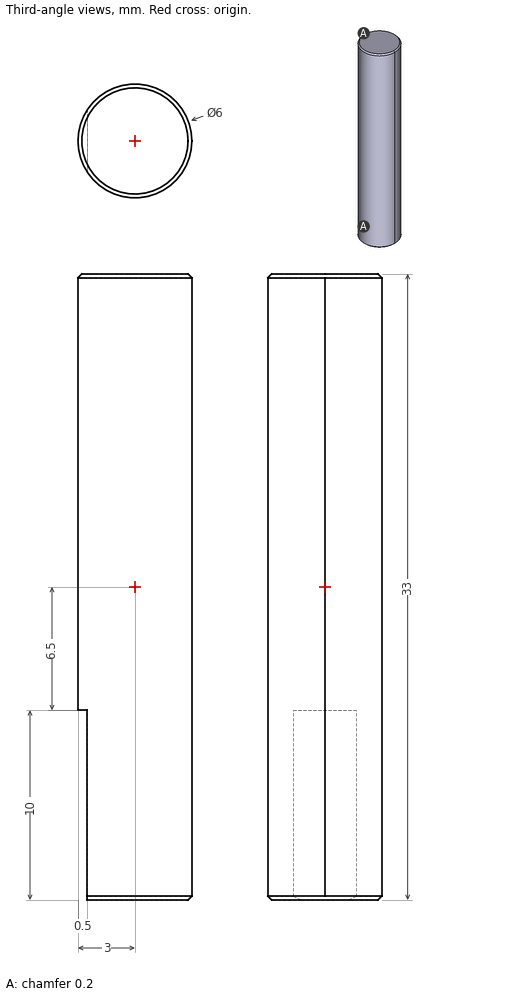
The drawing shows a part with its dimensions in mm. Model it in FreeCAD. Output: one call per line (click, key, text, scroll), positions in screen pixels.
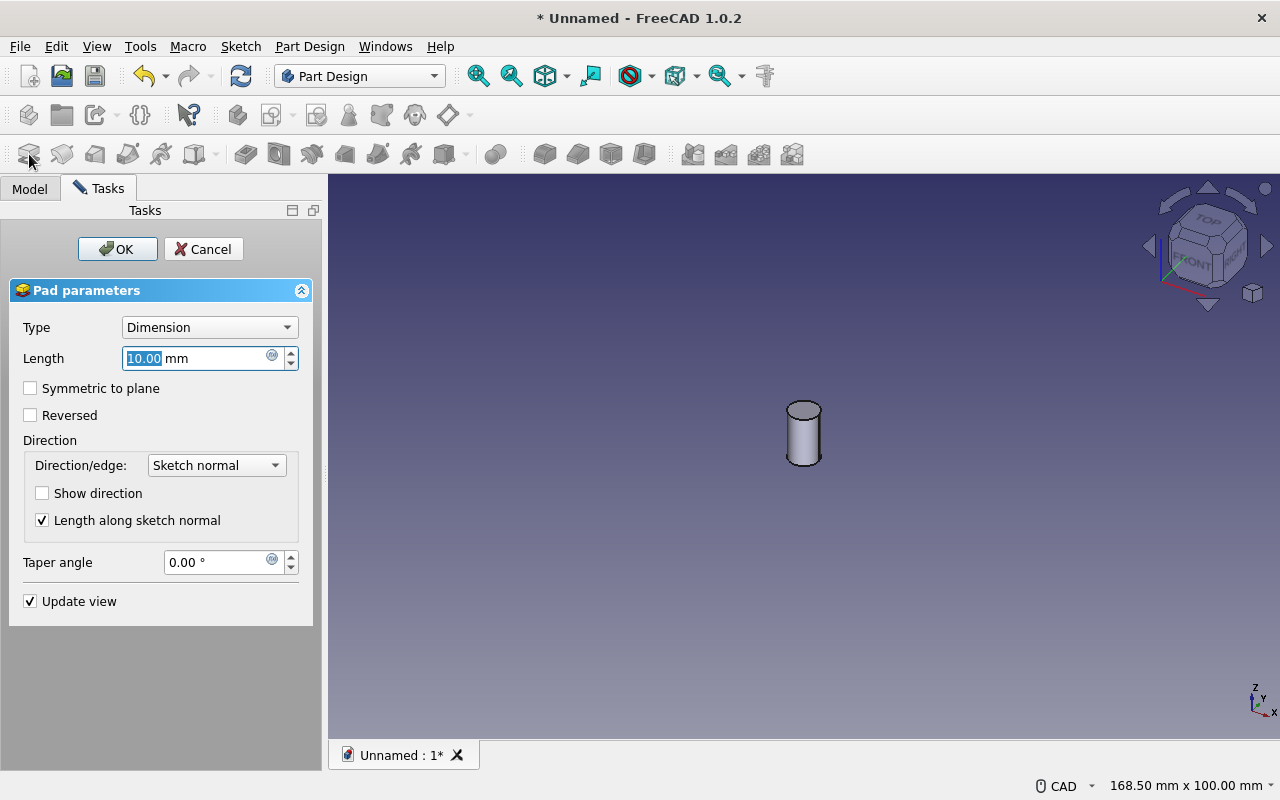
text(33)
key(Tab)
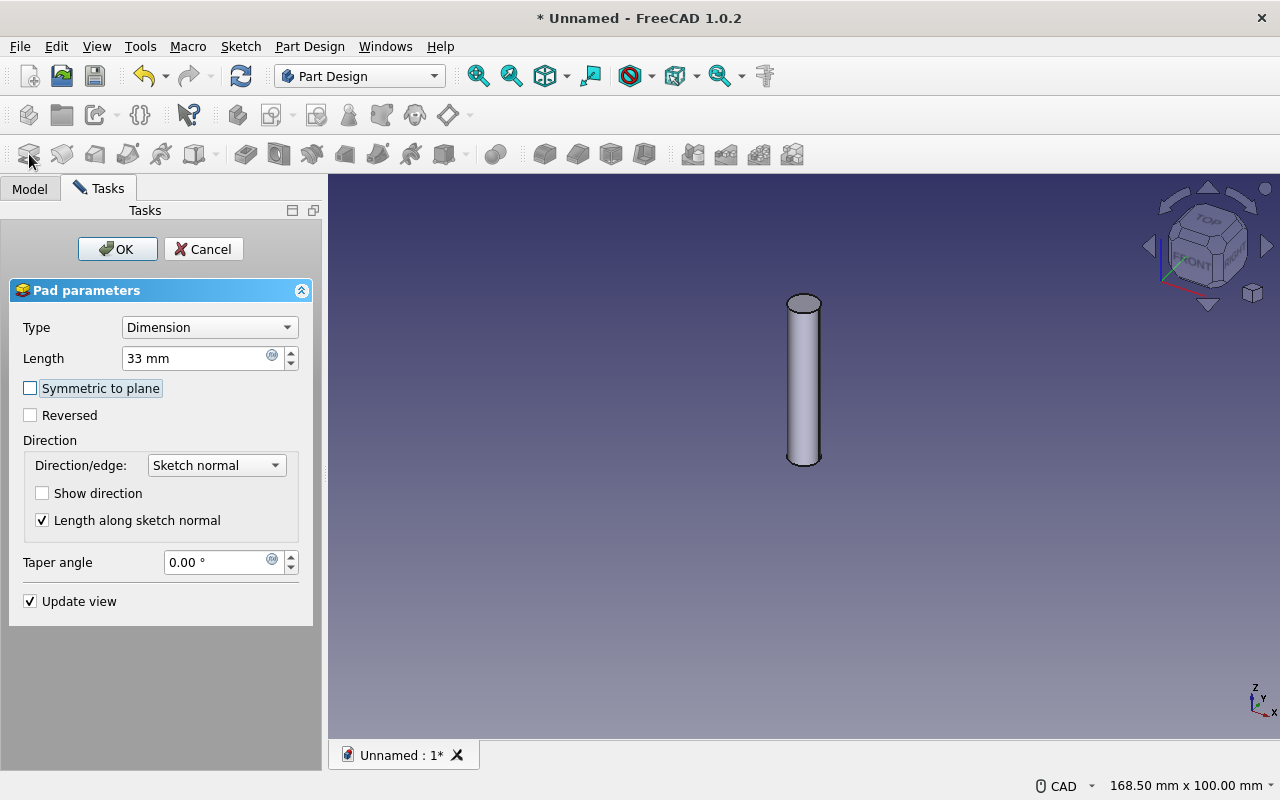
click(31, 388)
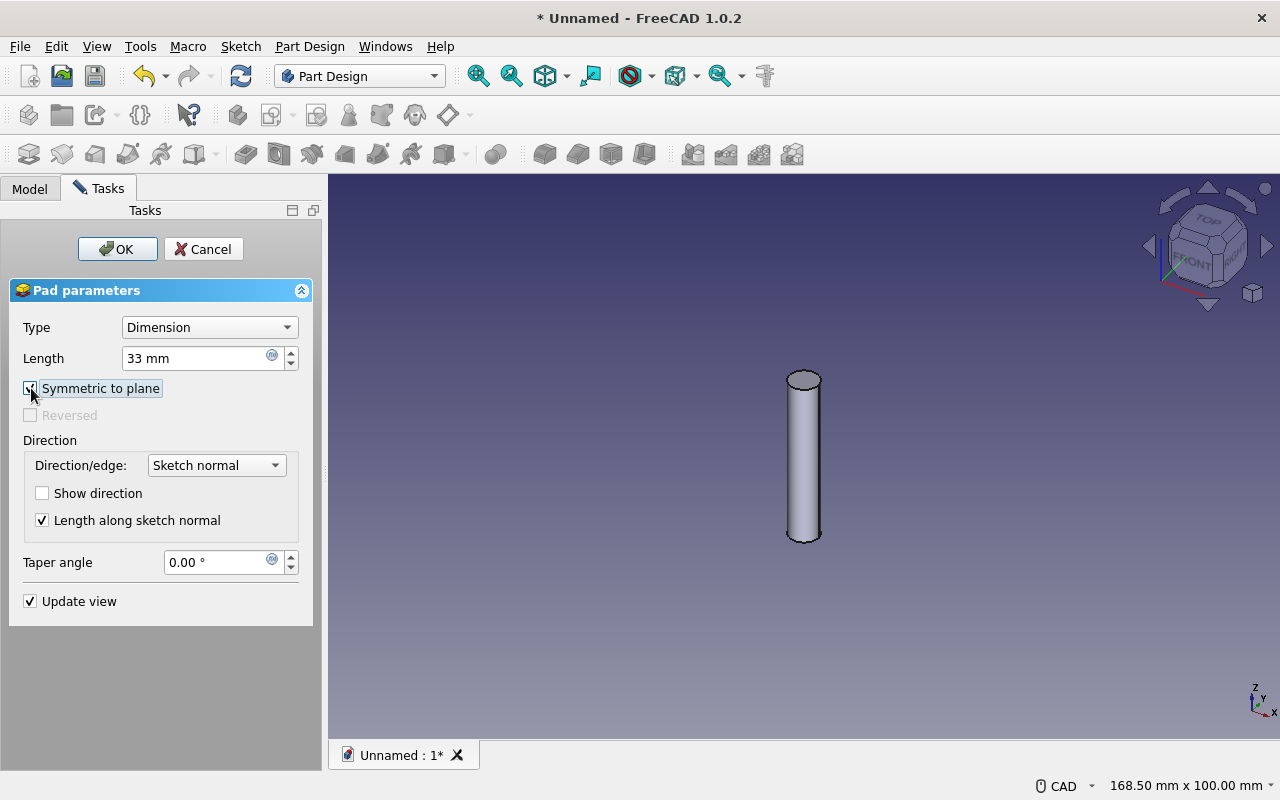
click(118, 249)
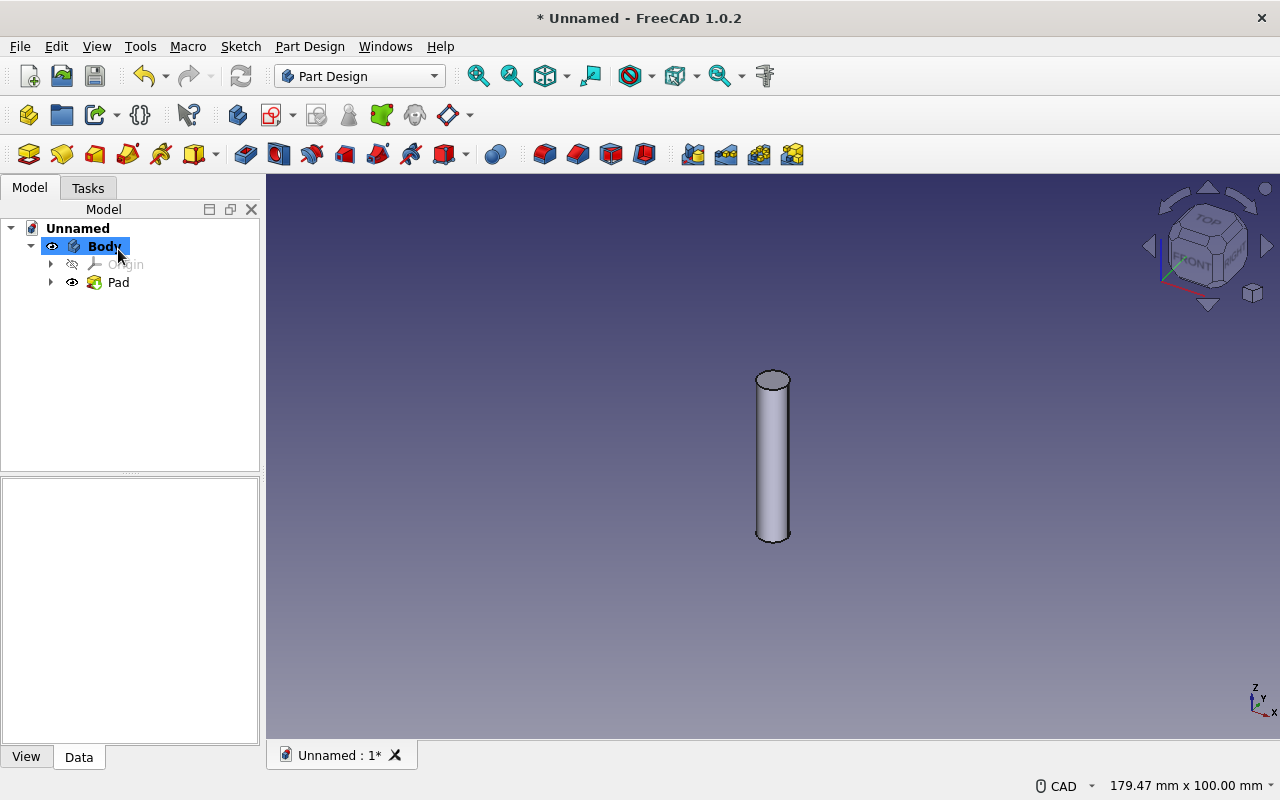
click(479, 76)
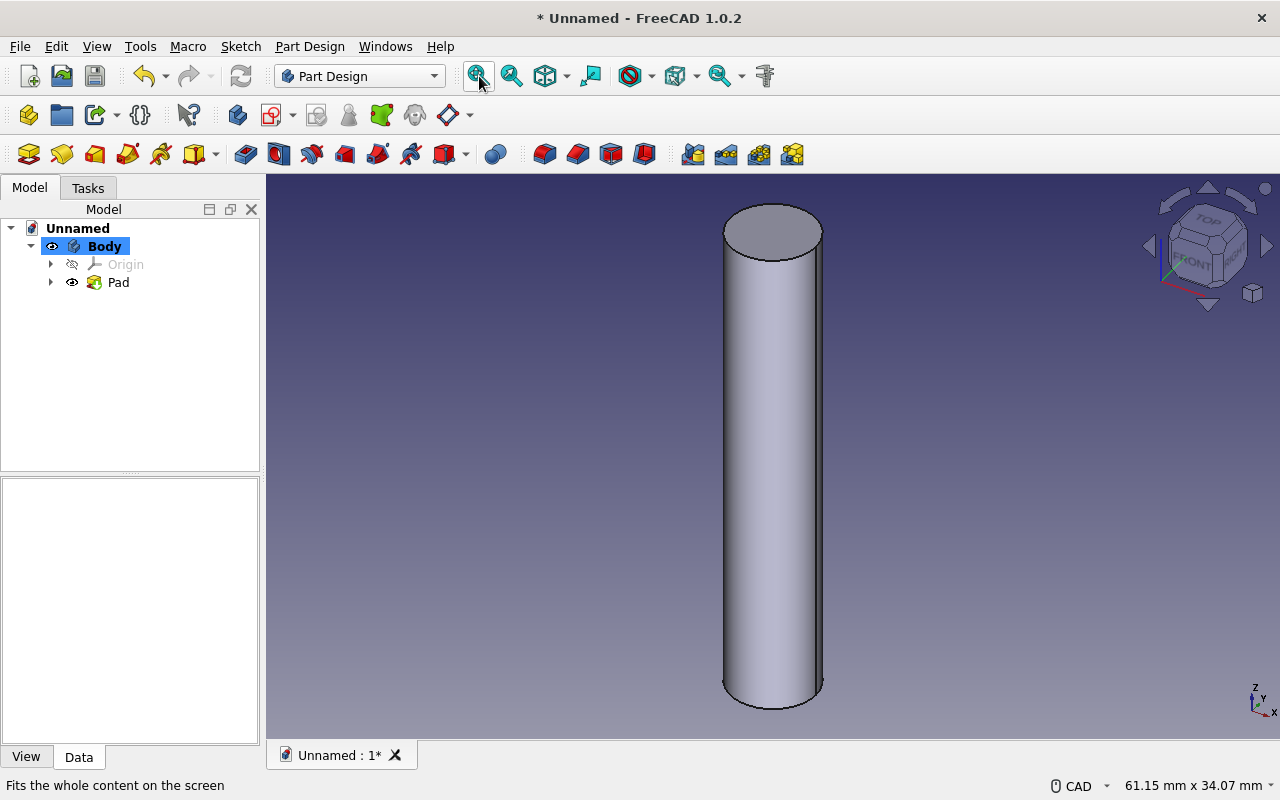
click(736, 699)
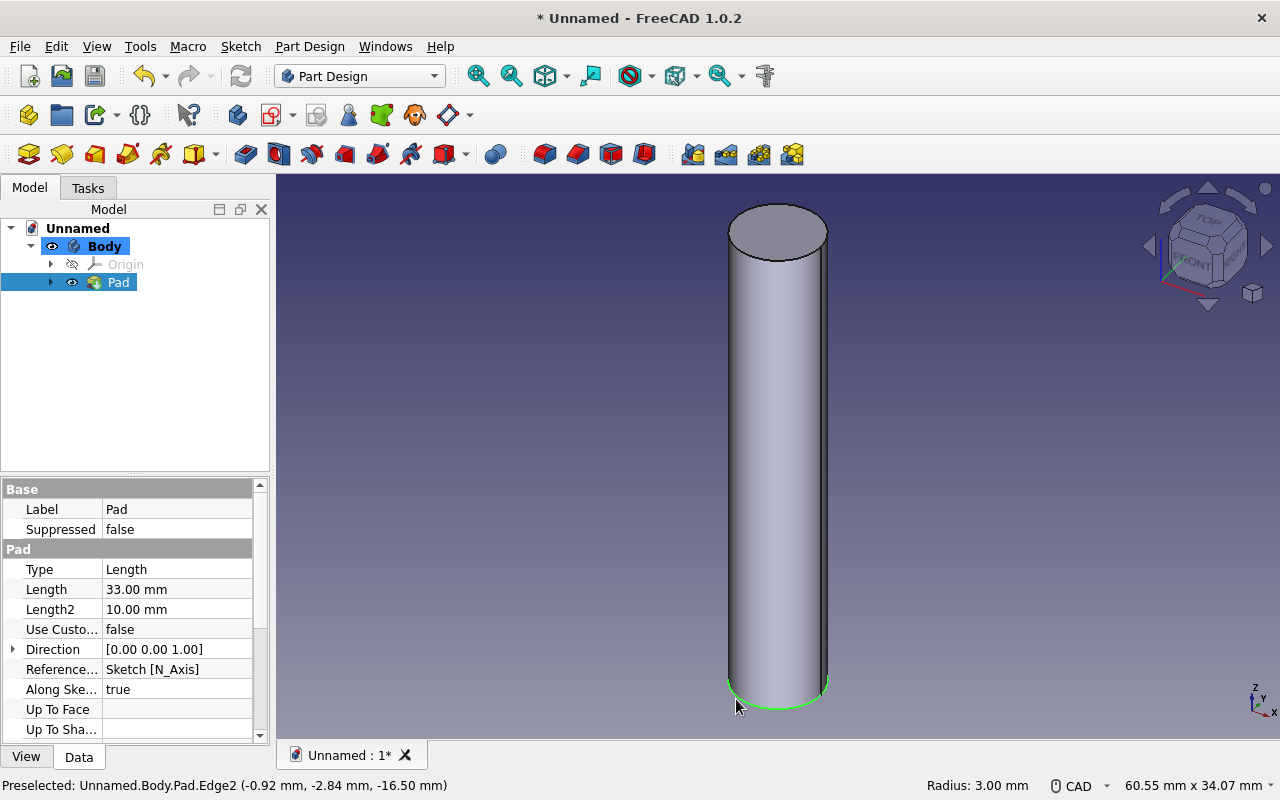
click(729, 234, ctrl)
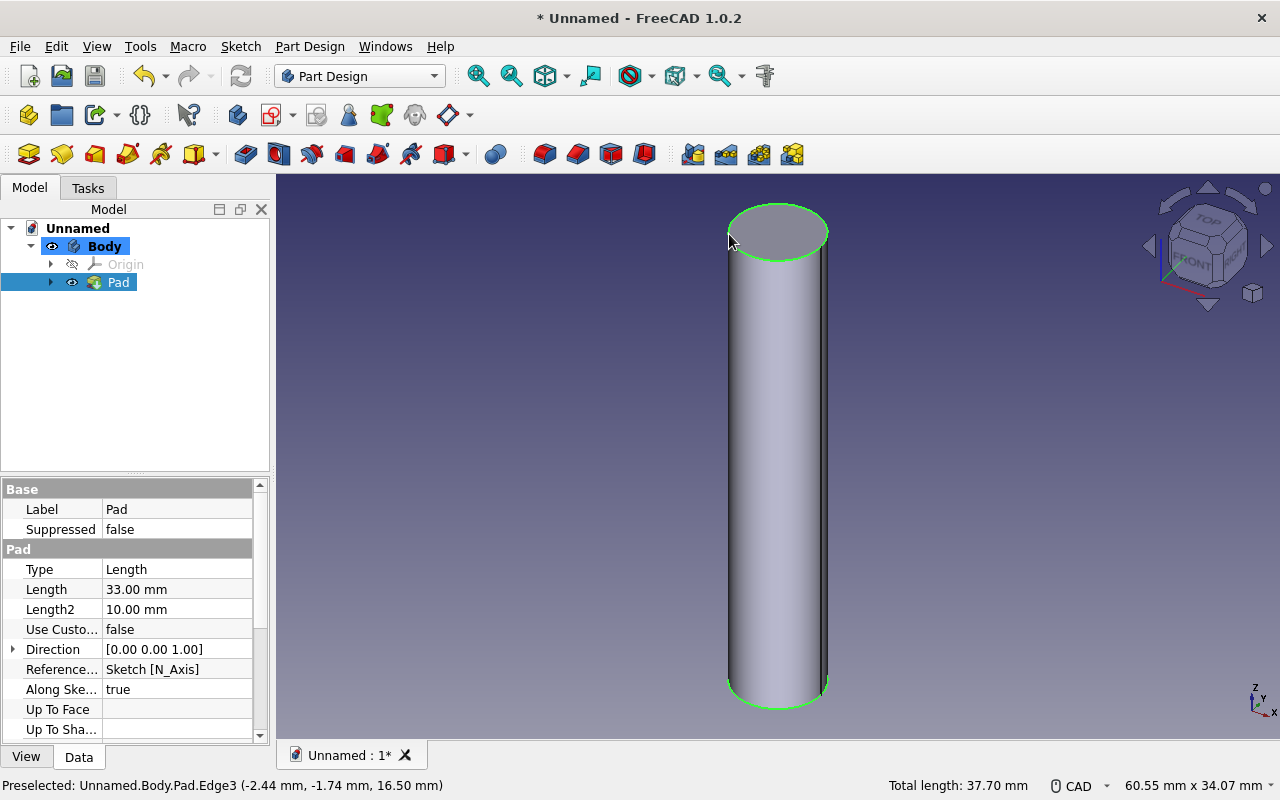
click(578, 154)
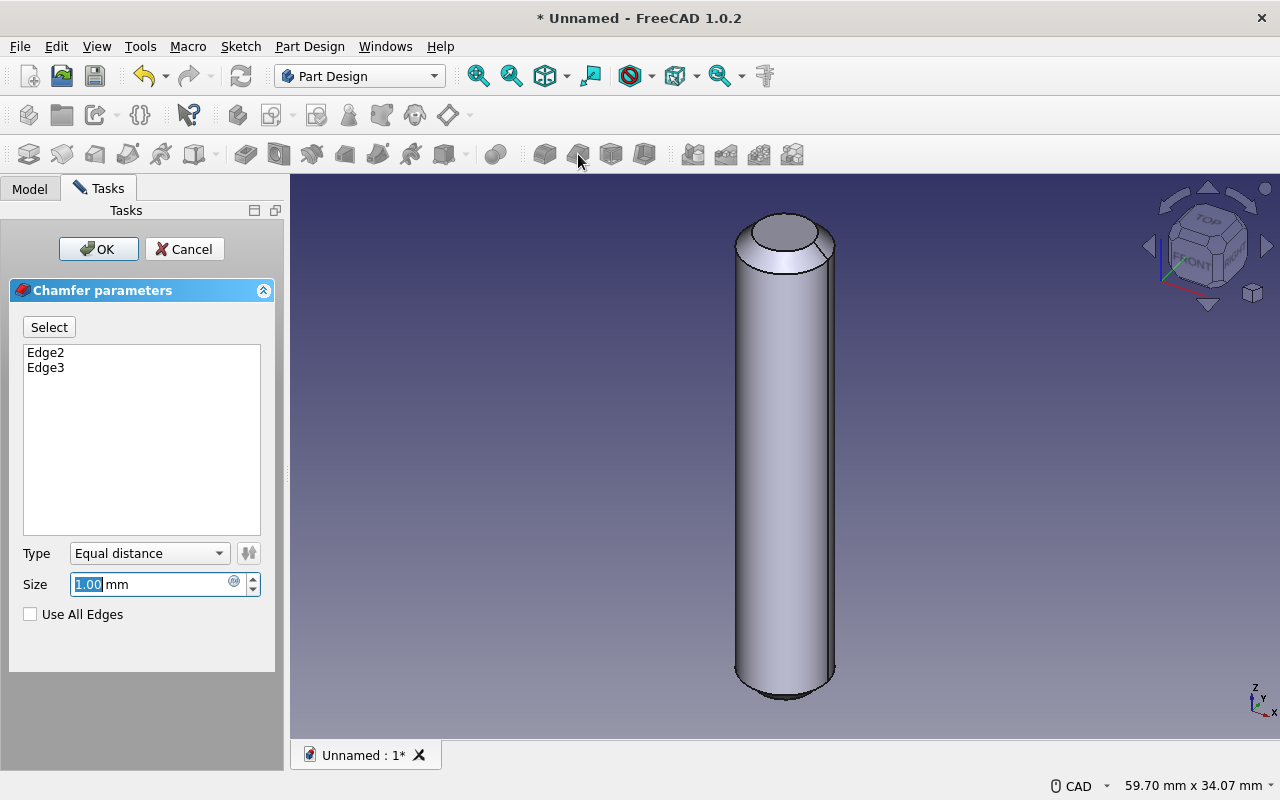
text(0.2)
key(Tab)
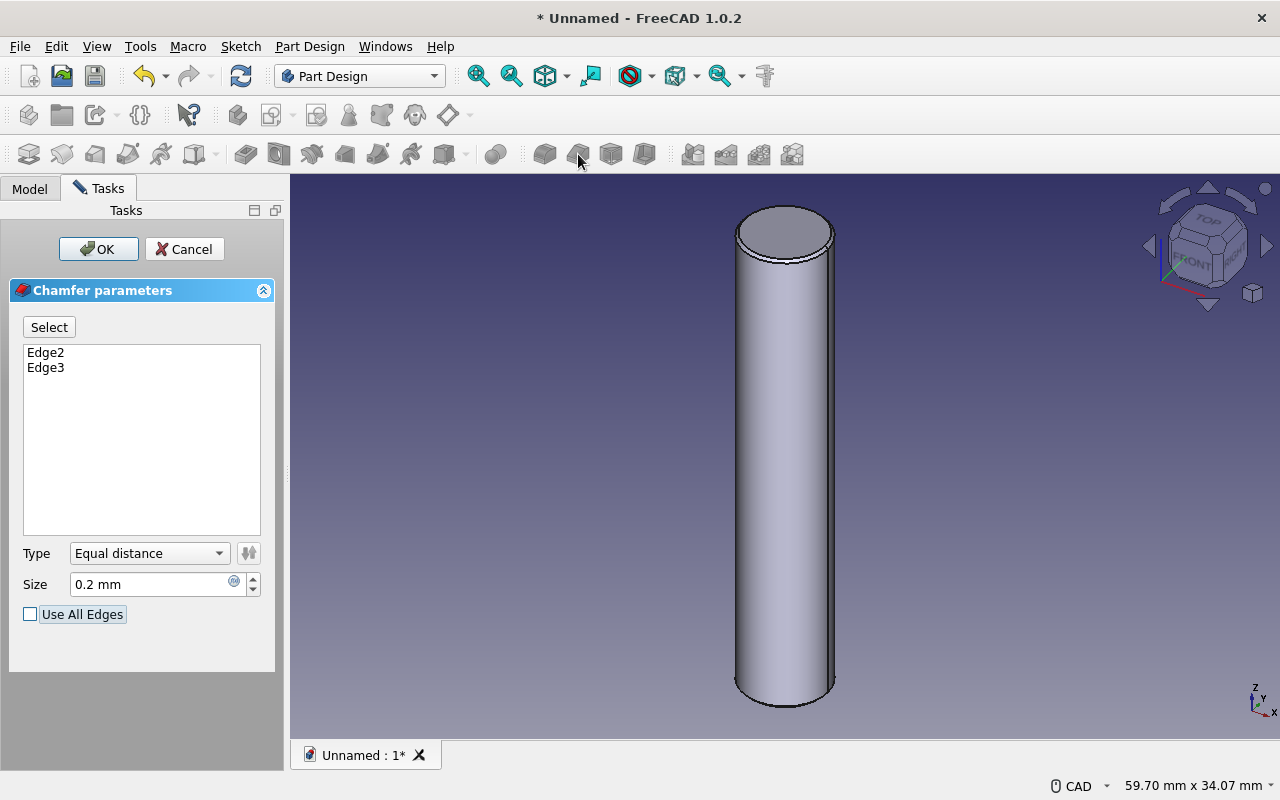
click(99, 249)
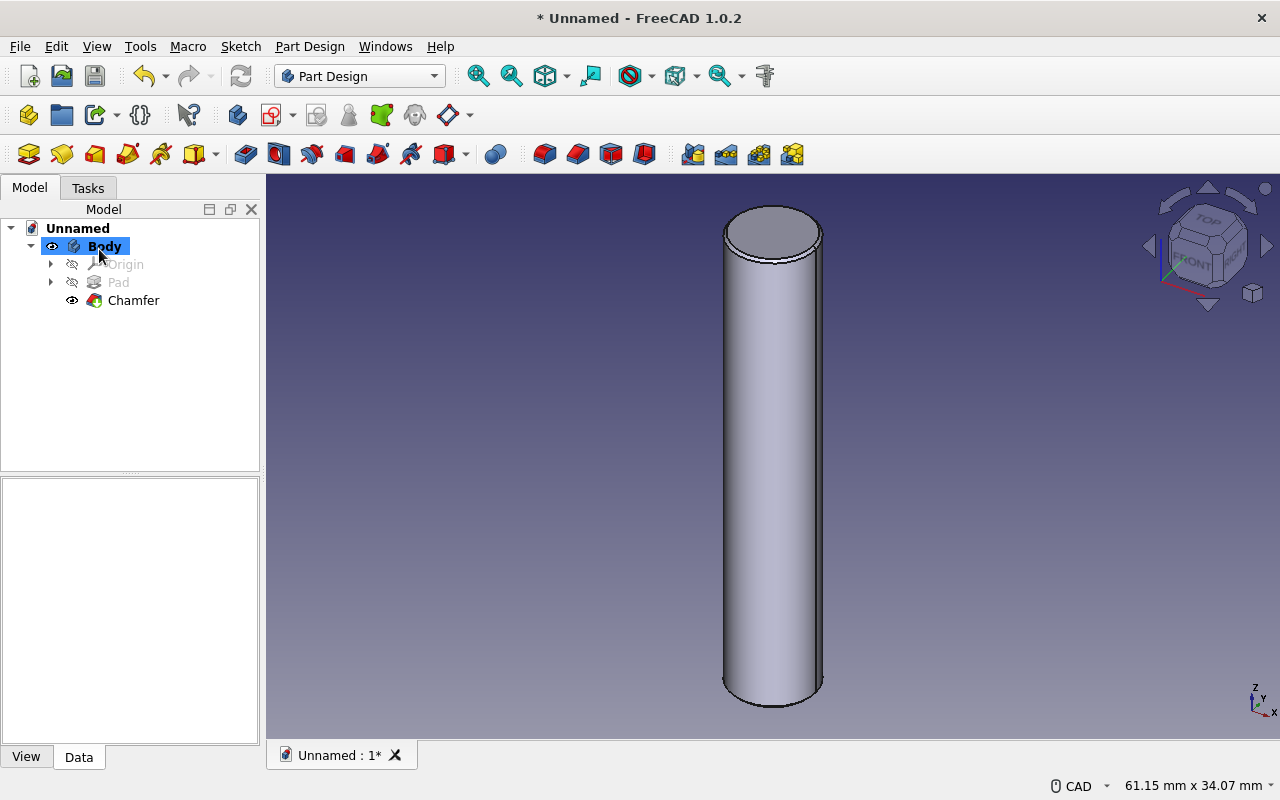
click(270, 116)